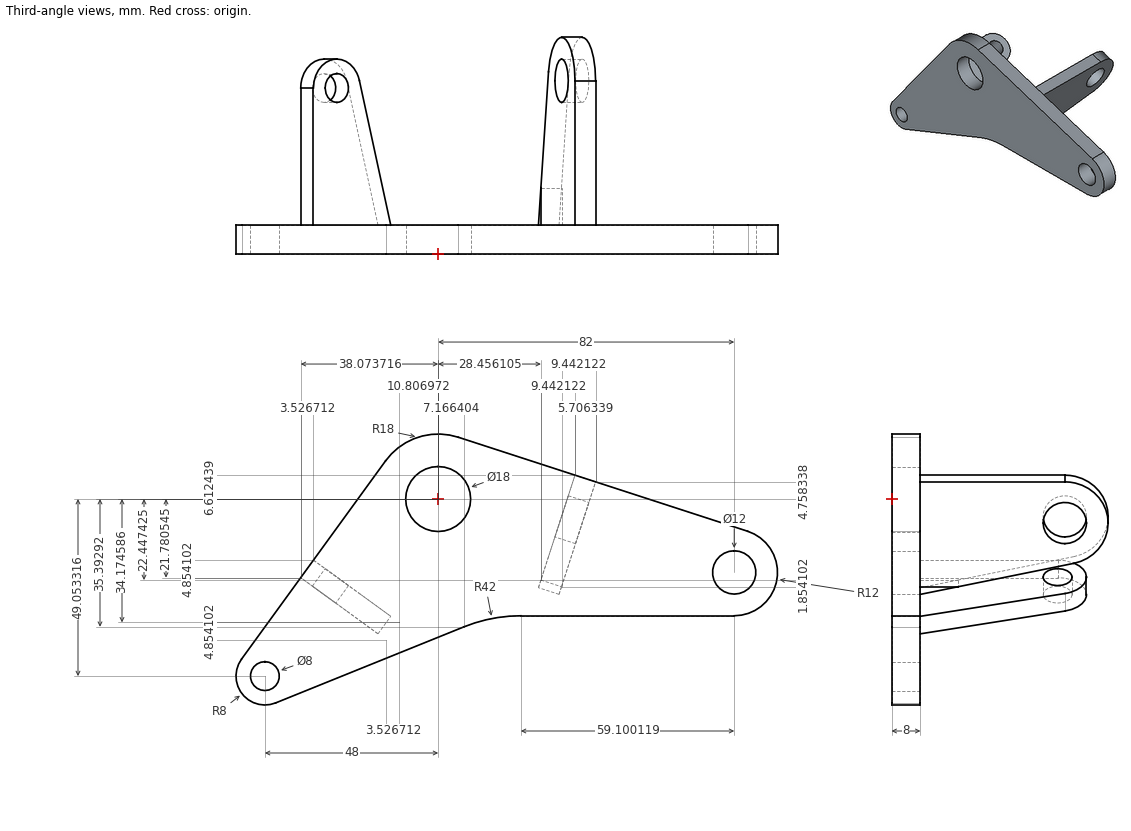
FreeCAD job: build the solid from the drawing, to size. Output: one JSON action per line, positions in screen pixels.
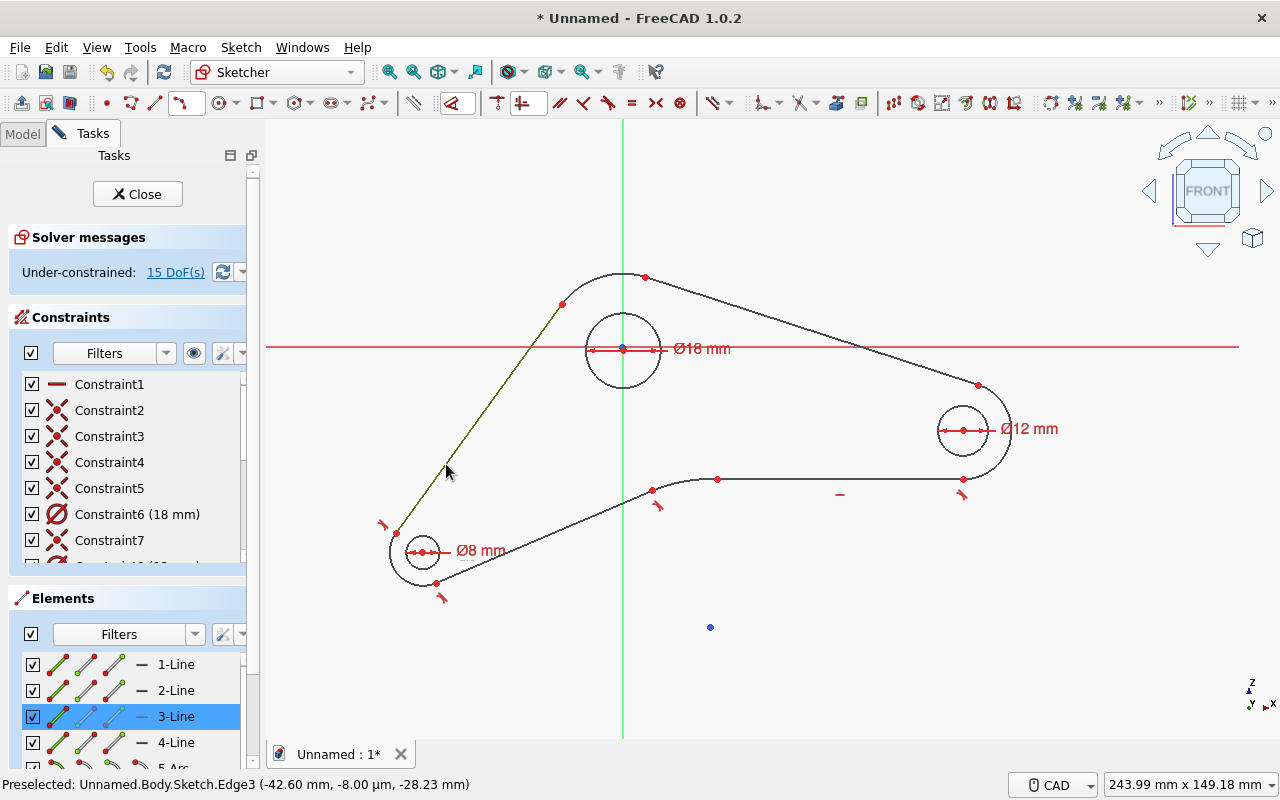
{"action": "left_click", "coordinate": [583, 285]}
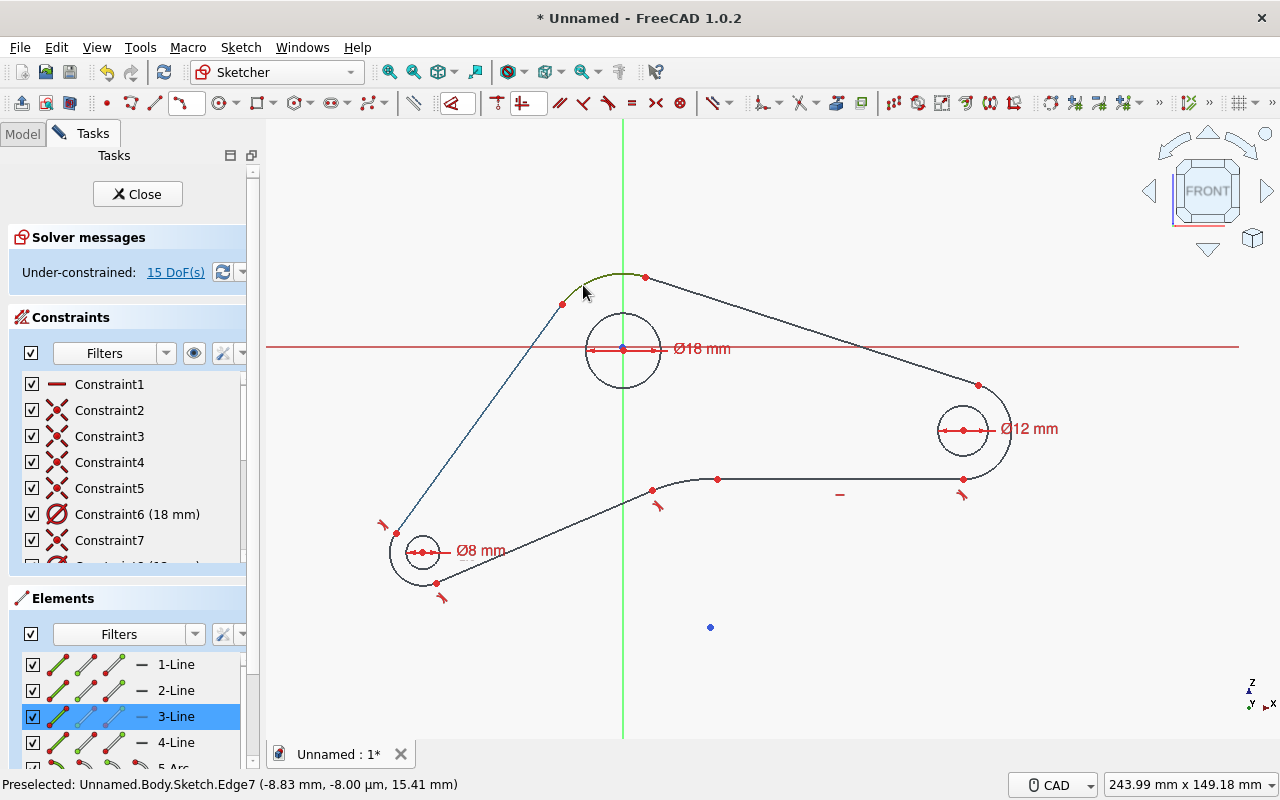
{"action": "key", "text": "t"}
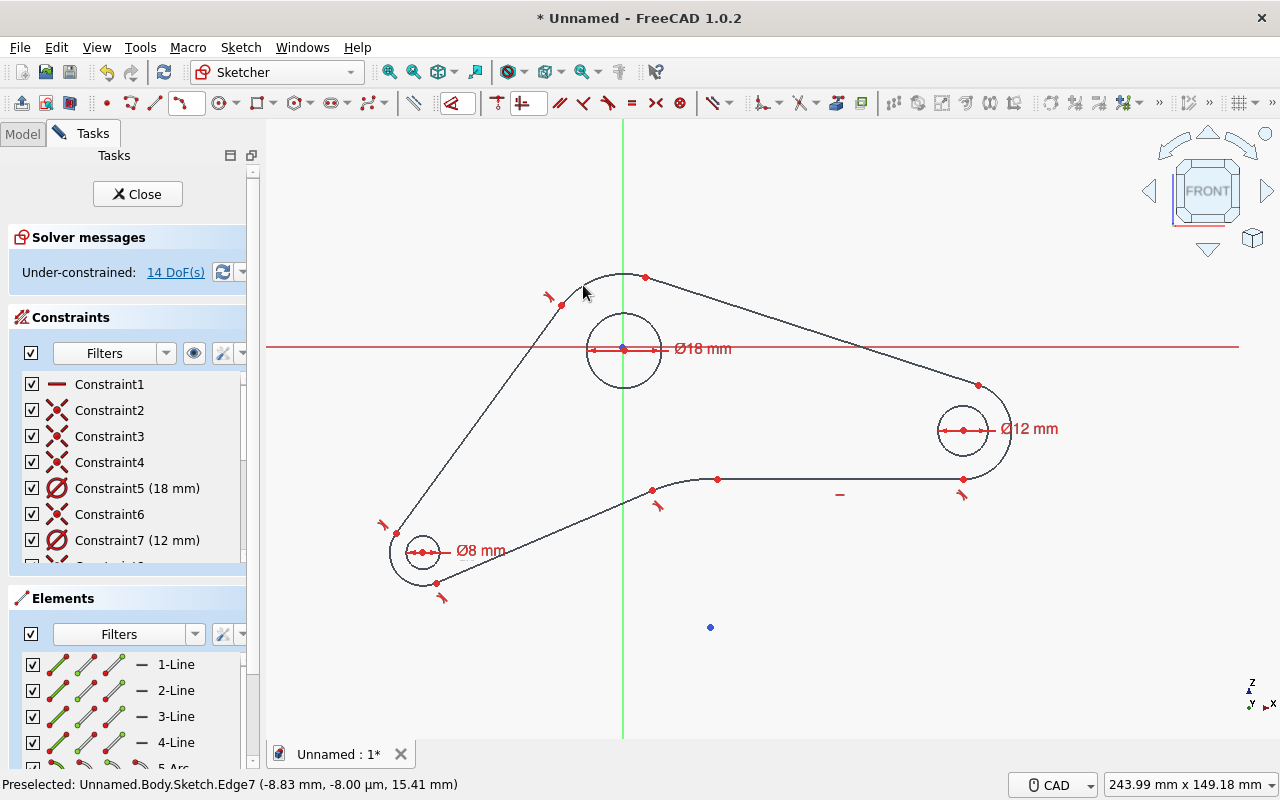
{"action": "left_click", "coordinate": [746, 310]}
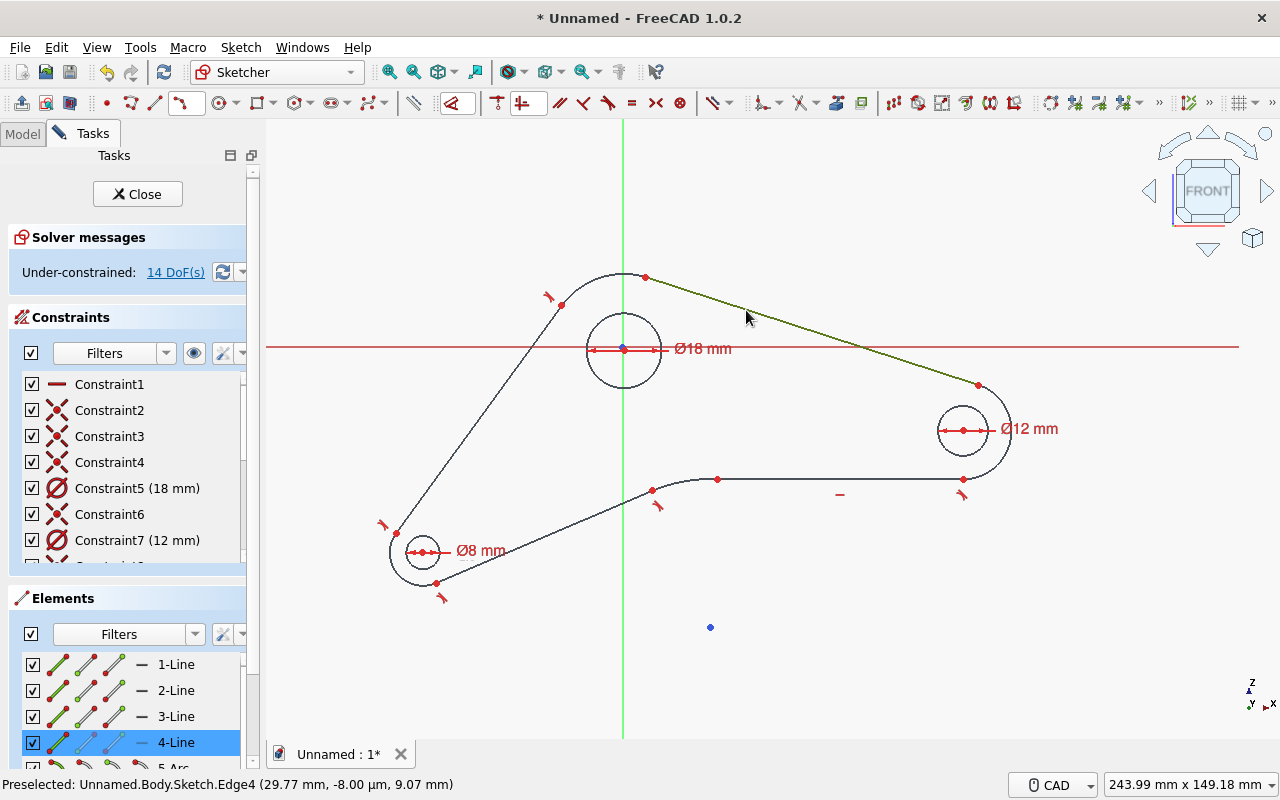
{"action": "left_click", "coordinate": [583, 286]}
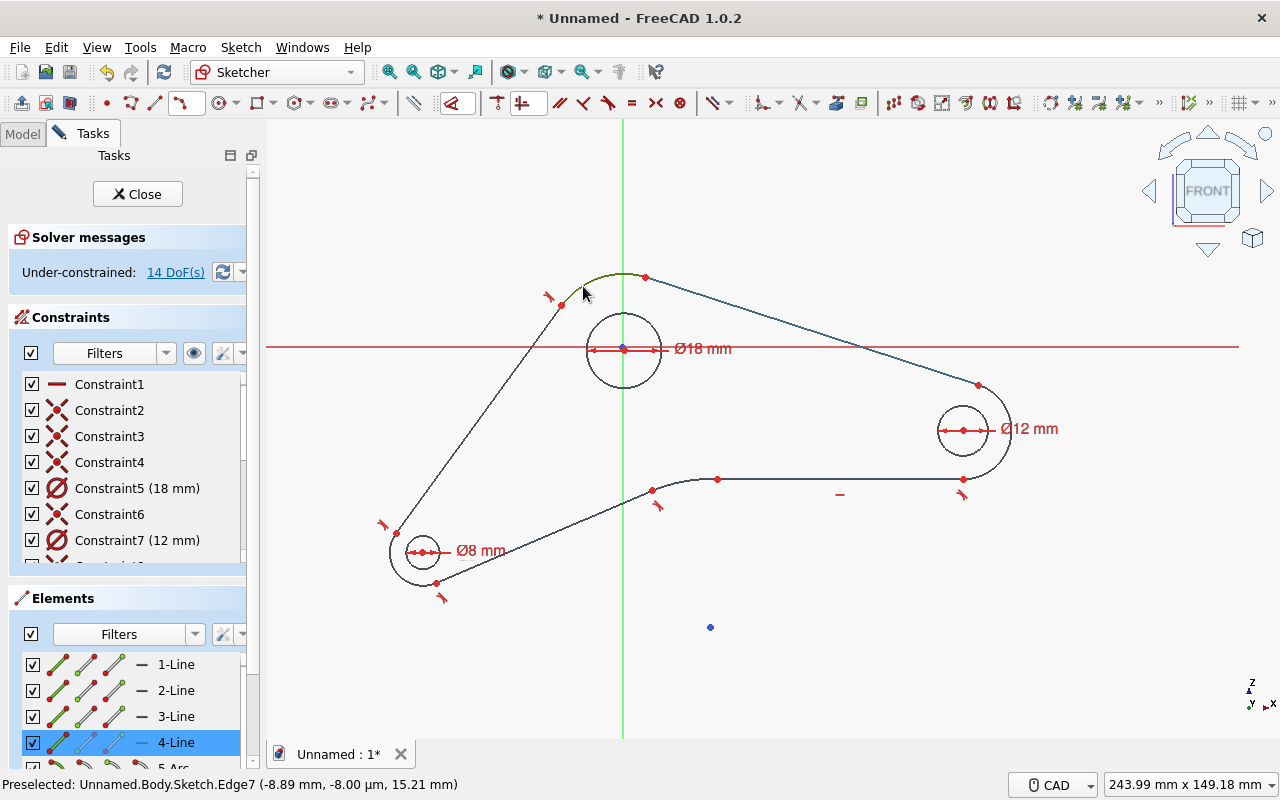
{"action": "left_click", "coordinate": [608, 104]}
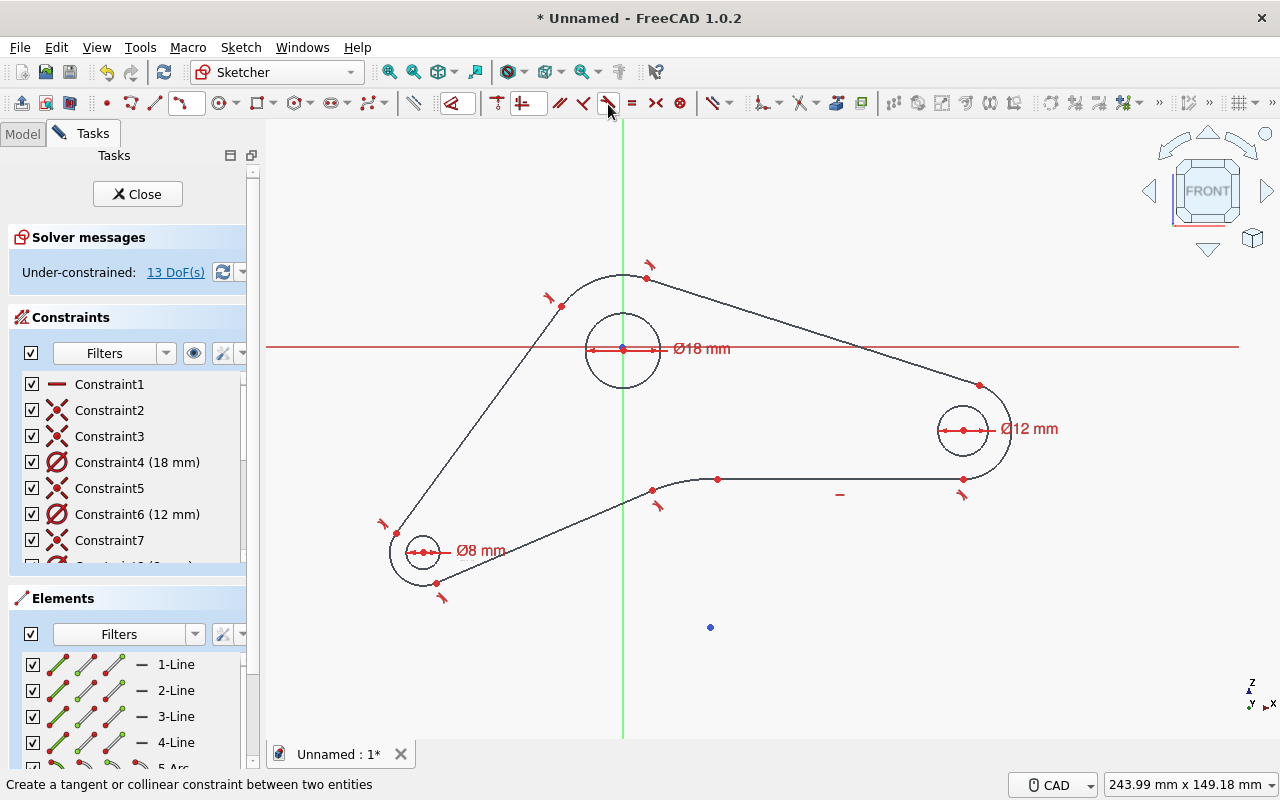
{"action": "left_click", "coordinate": [746, 311]}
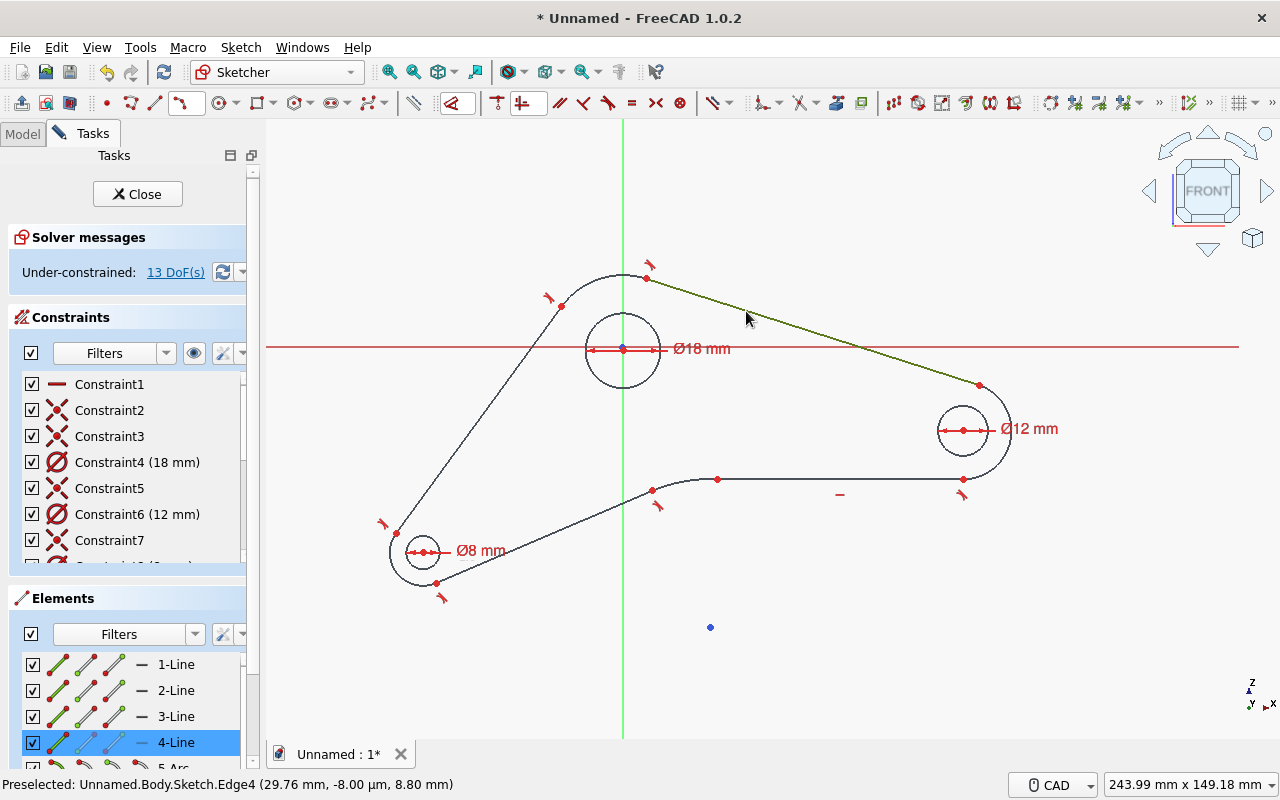
{"action": "left_click", "coordinate": [999, 463]}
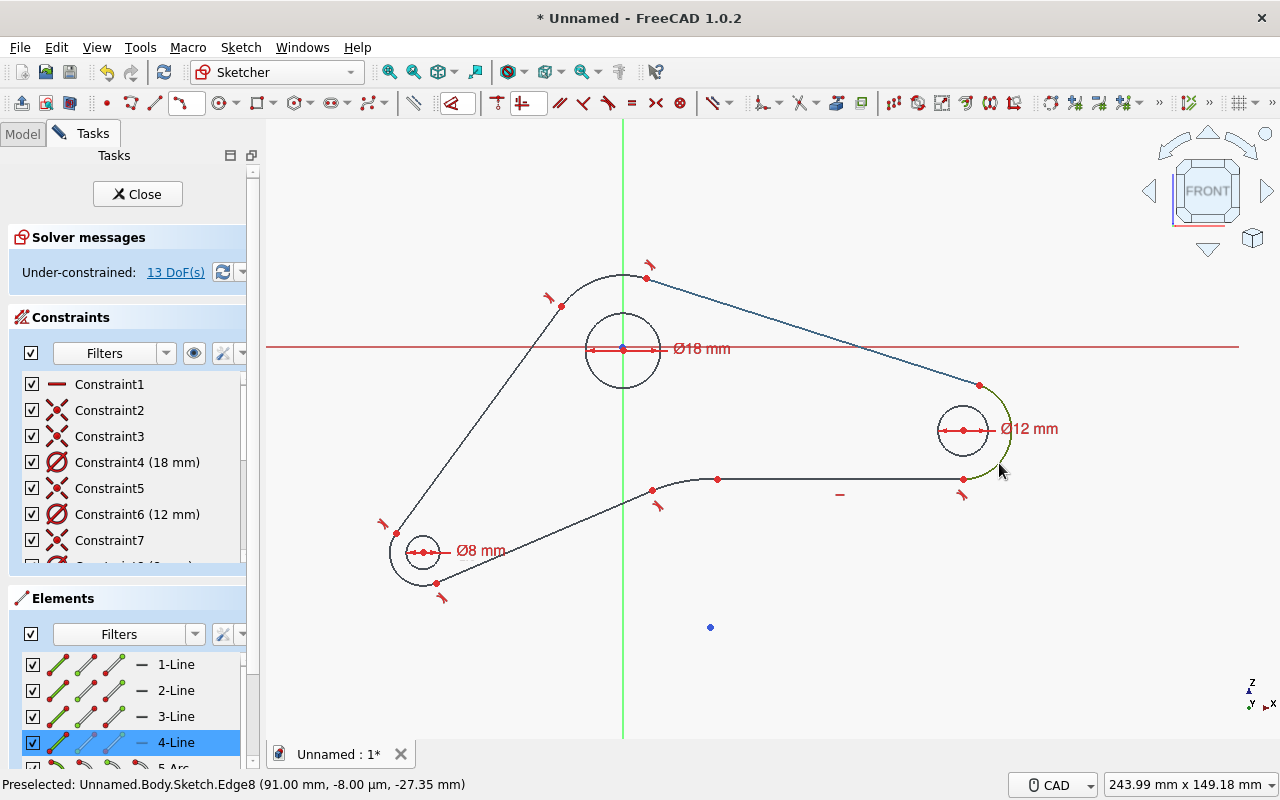
{"action": "left_click", "coordinate": [608, 104]}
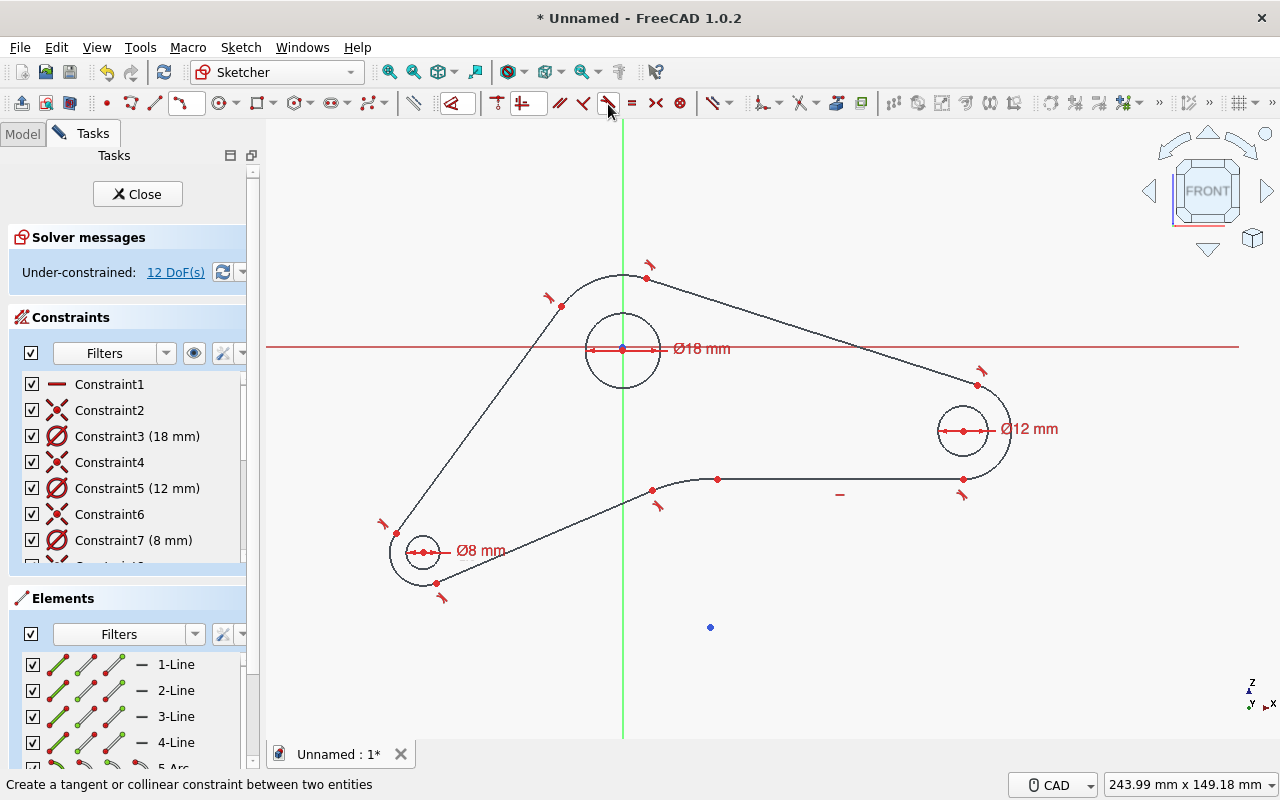
{"action": "scroll", "coordinate": [623, 349], "scroll_direction": "up", "scroll_amount": 5}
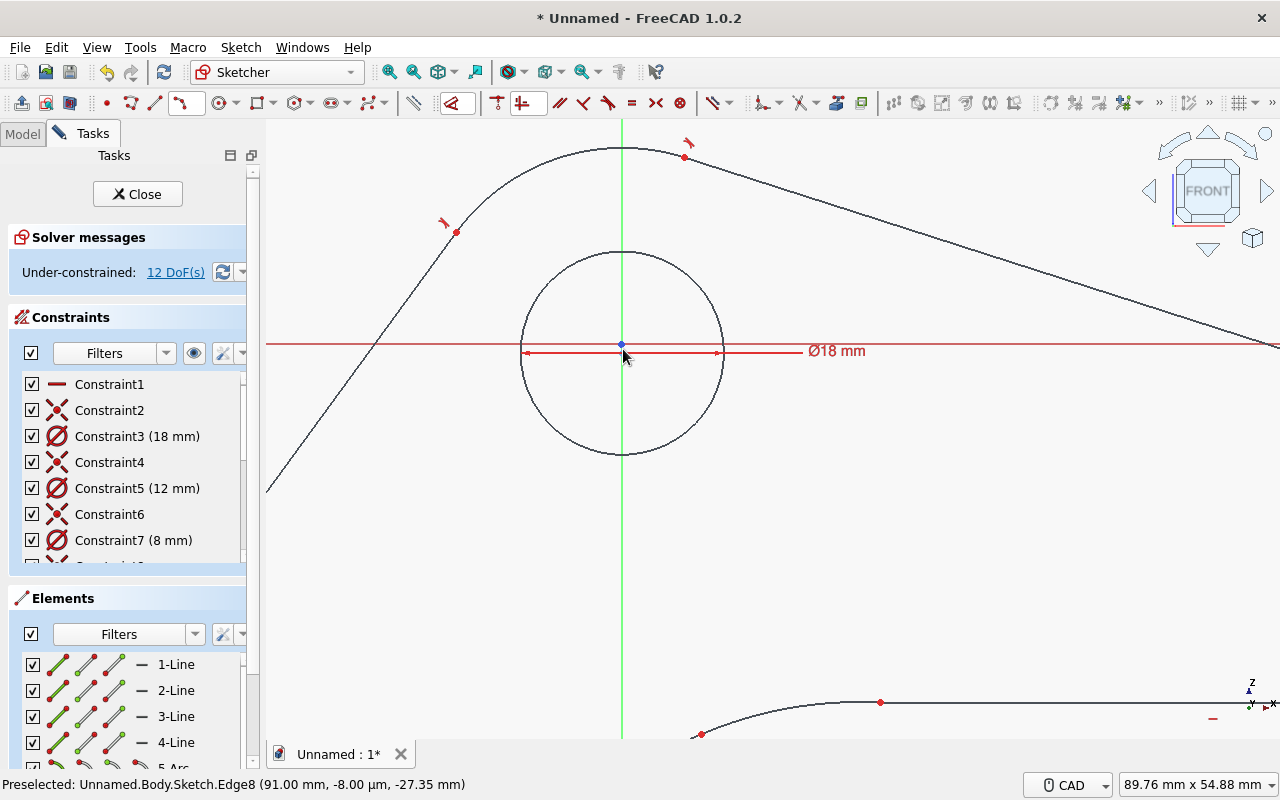
{"action": "left_click_drag", "start_coordinate": [612, 334], "coordinate": [632, 363]}